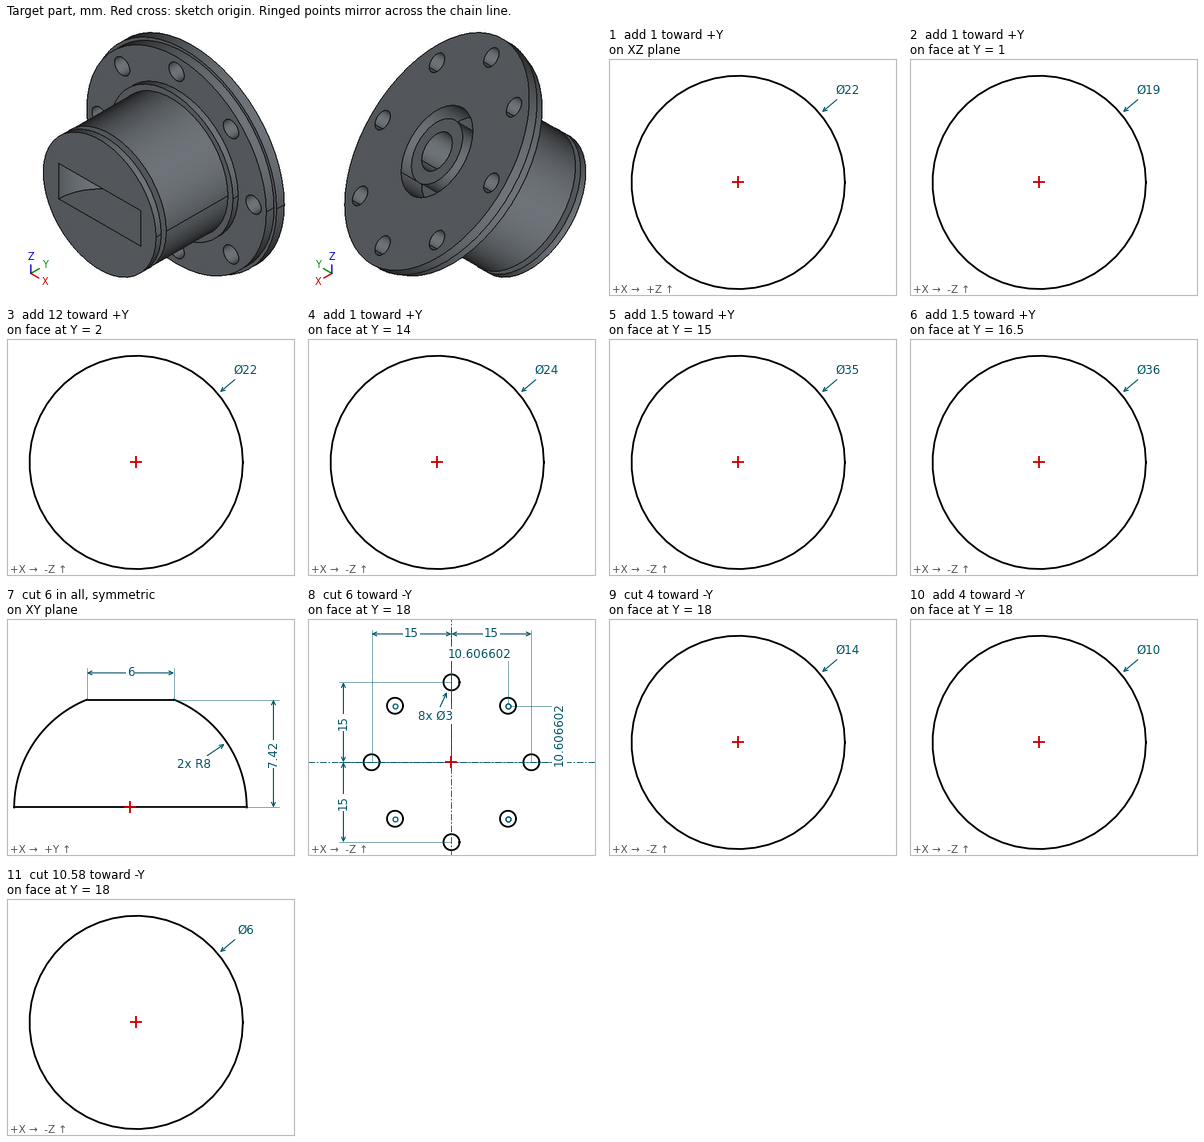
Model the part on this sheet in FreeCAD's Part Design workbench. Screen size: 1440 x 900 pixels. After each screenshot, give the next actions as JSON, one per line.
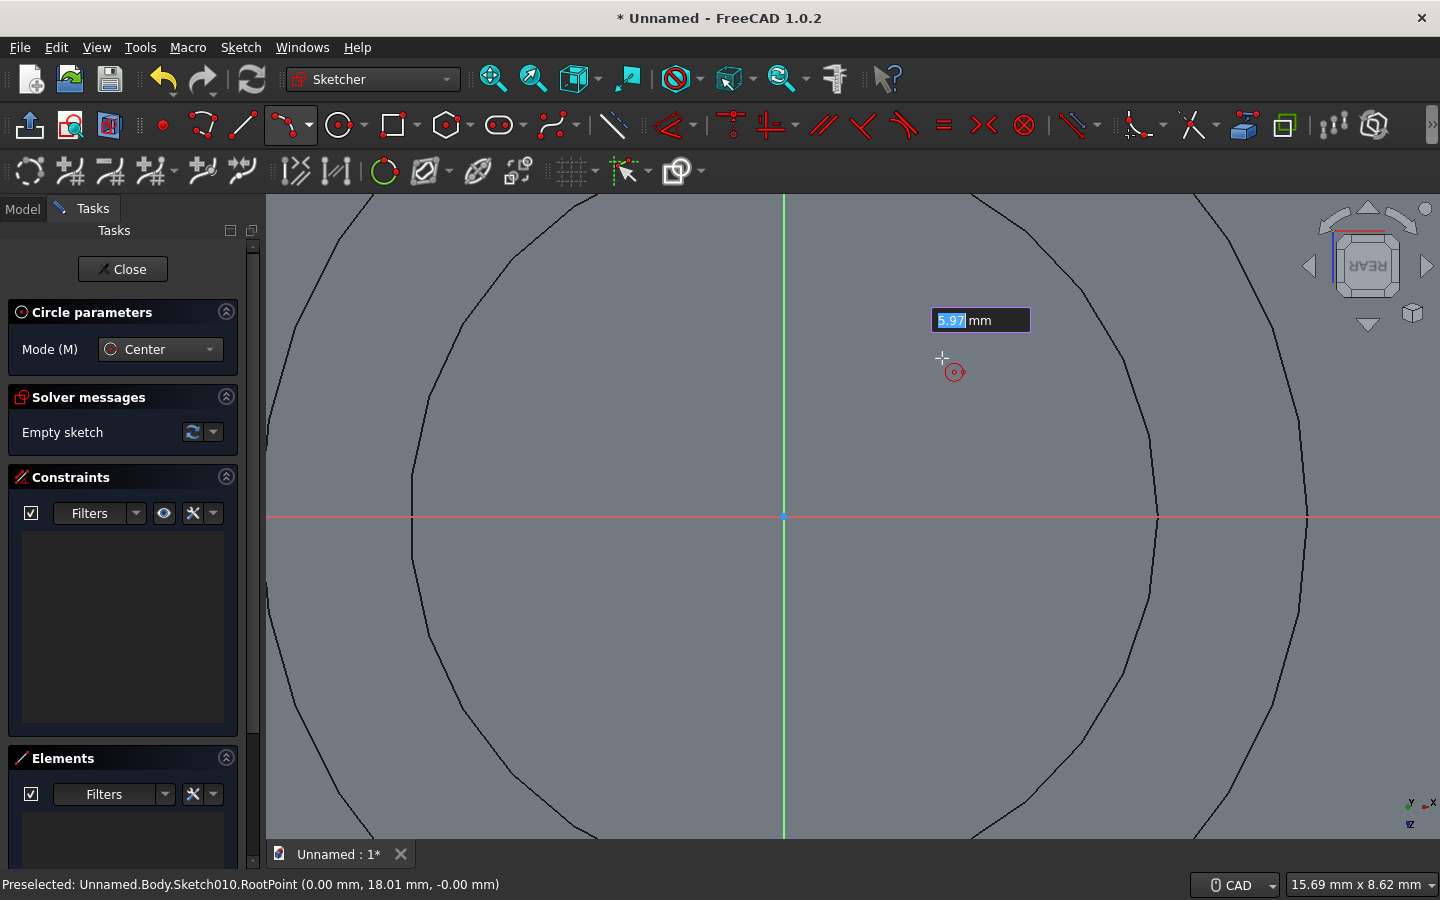
{"action": "type", "text": "6"}
{"action": "key", "text": "Return"}
{"action": "key", "text": "Escape"}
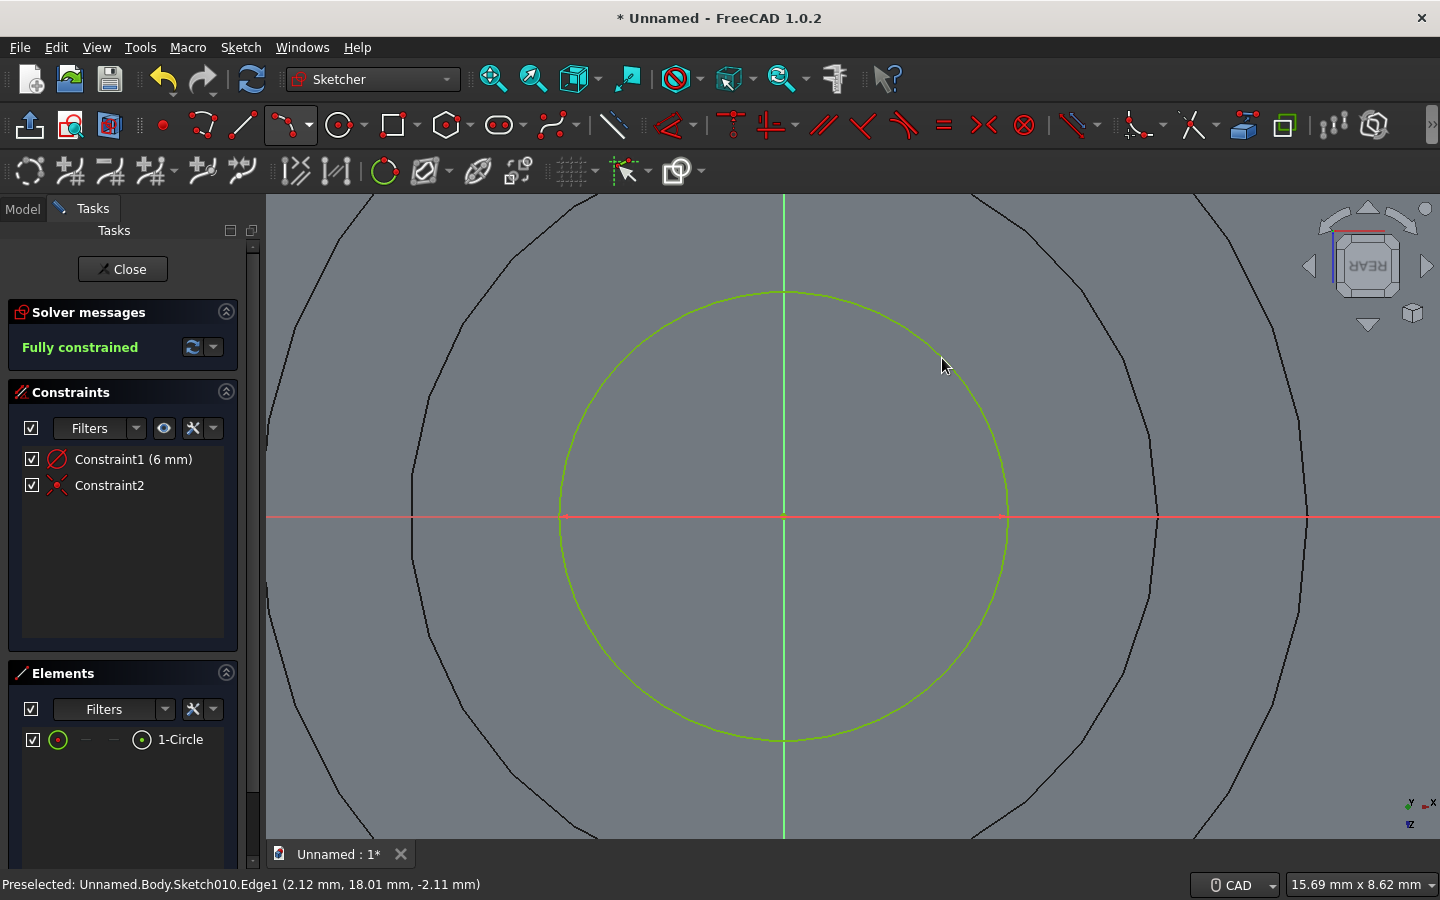
{"action": "left_click", "coordinate": [123, 269]}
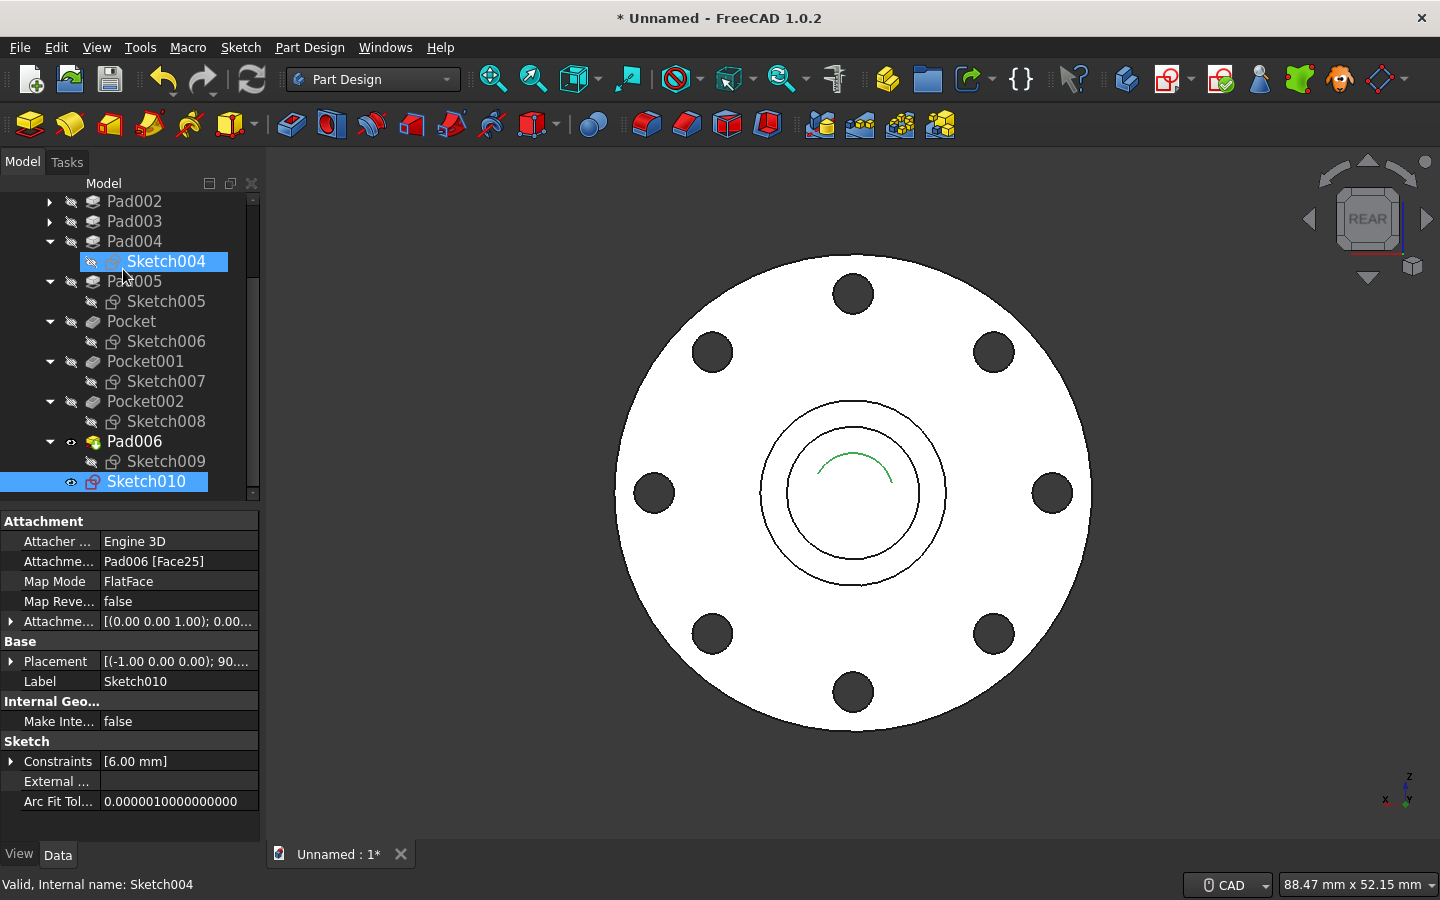
{"action": "left_click", "coordinate": [292, 124]}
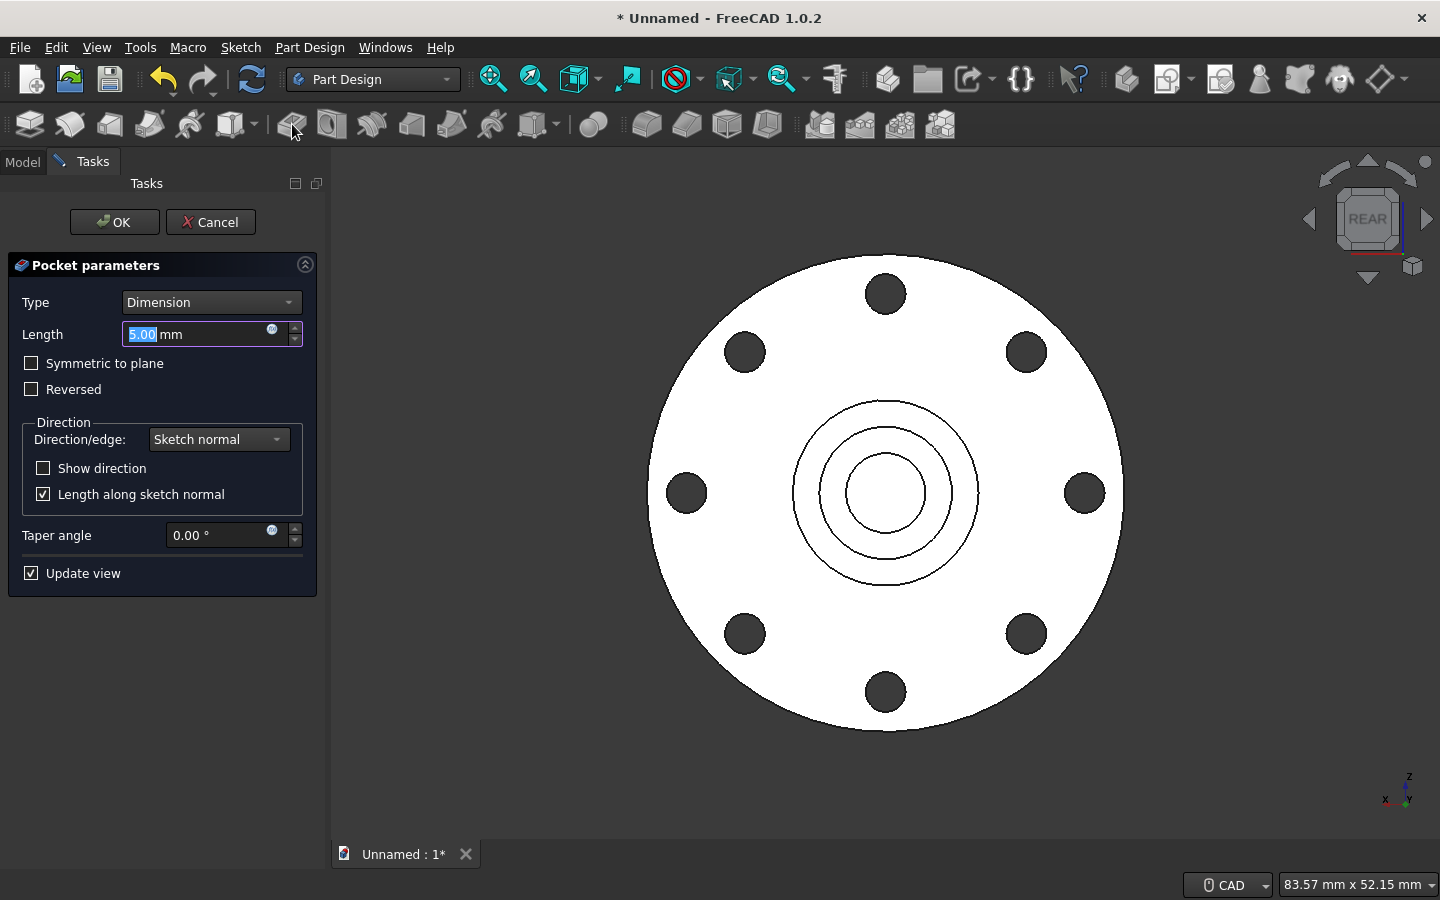
{"action": "type", "text": "10.58"}
{"action": "key", "text": "Tab"}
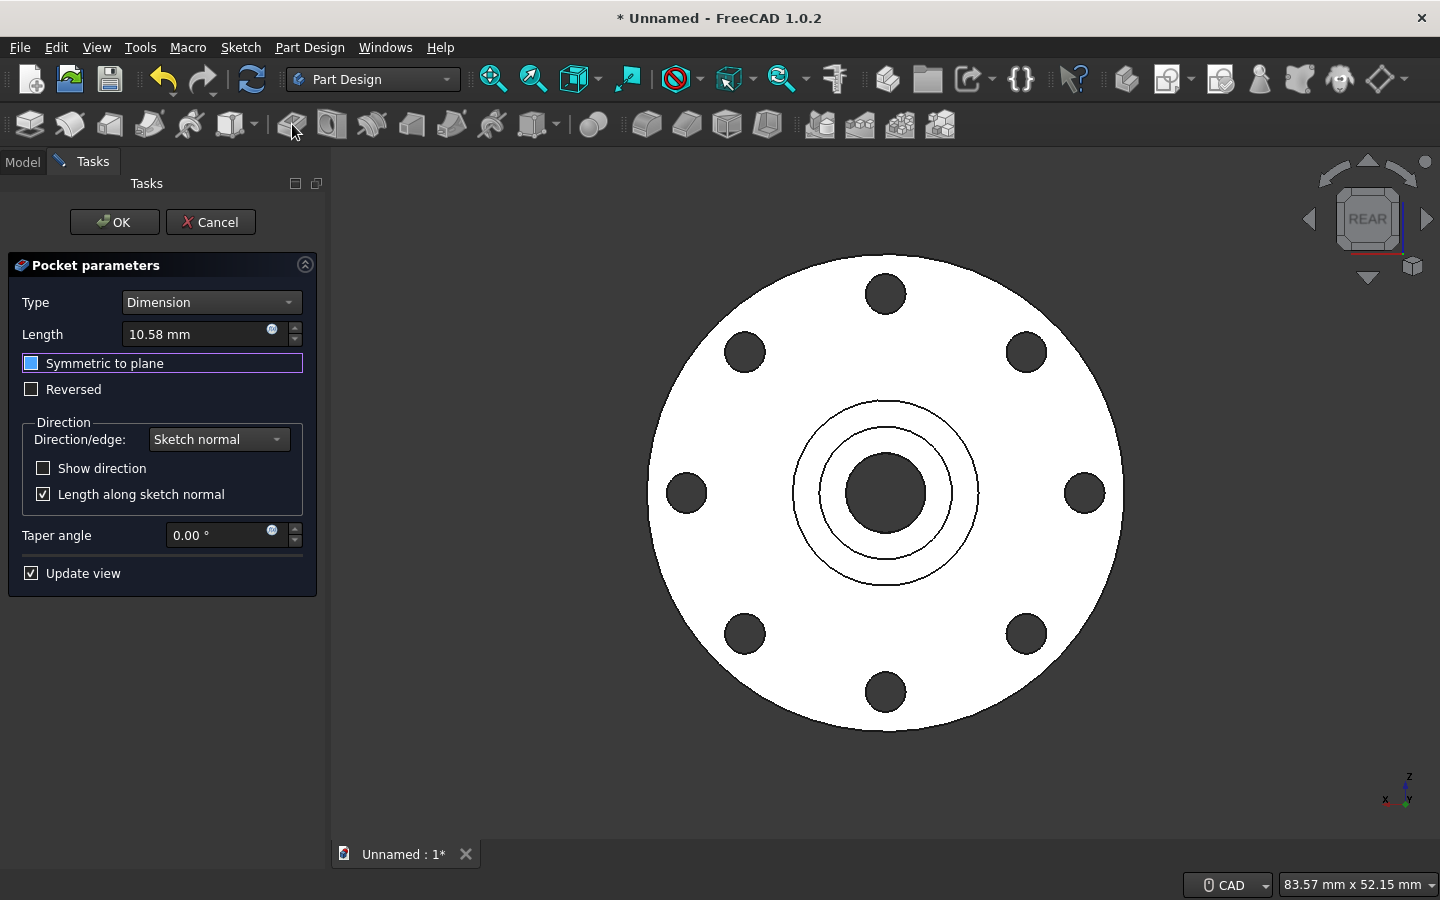
{"action": "left_click", "coordinate": [115, 222]}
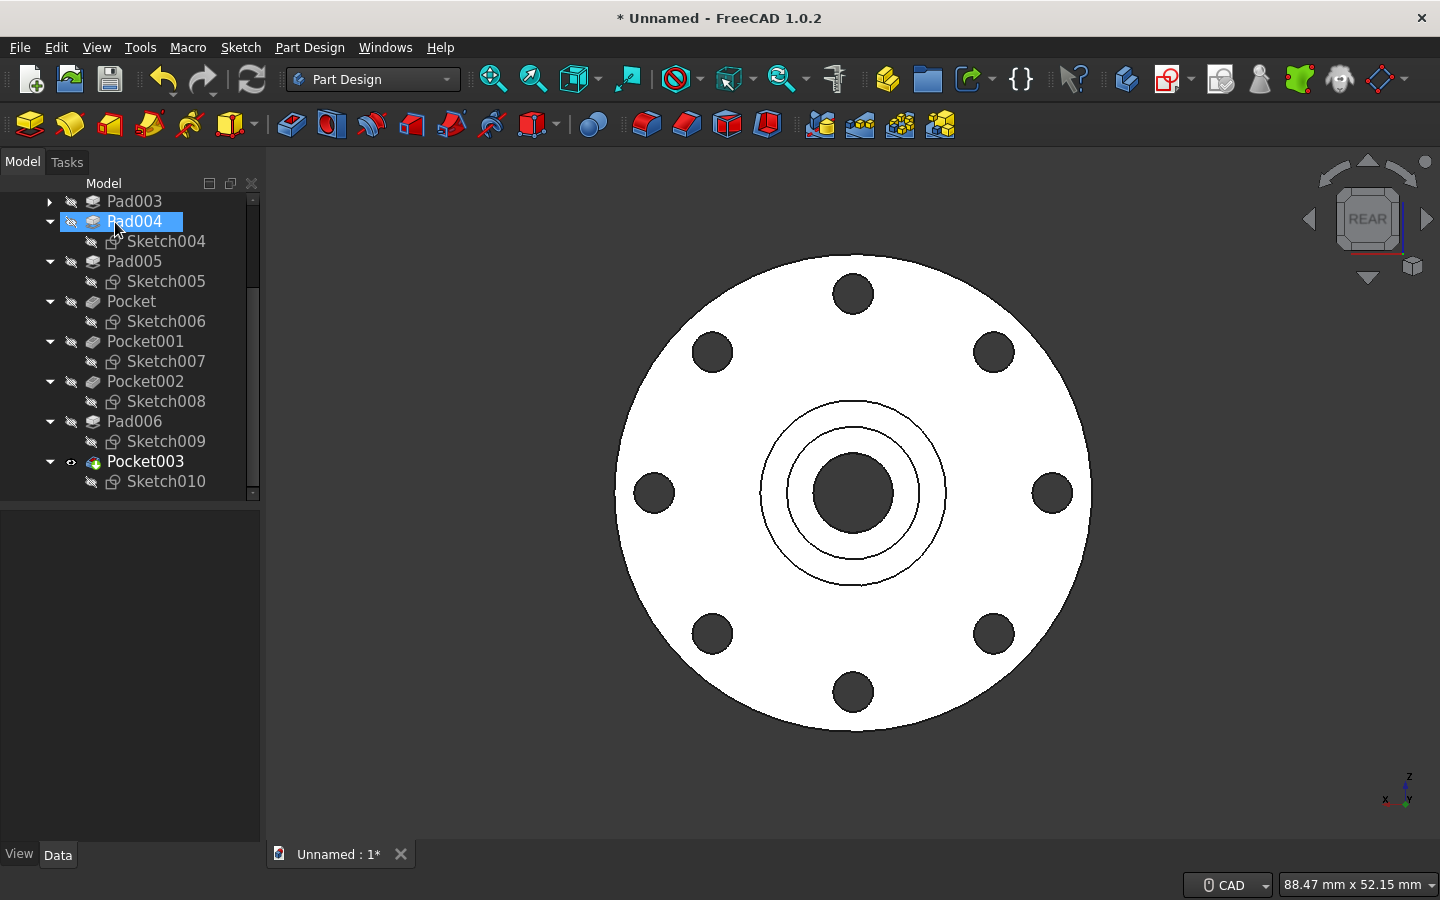
{"action": "key", "text": "0"}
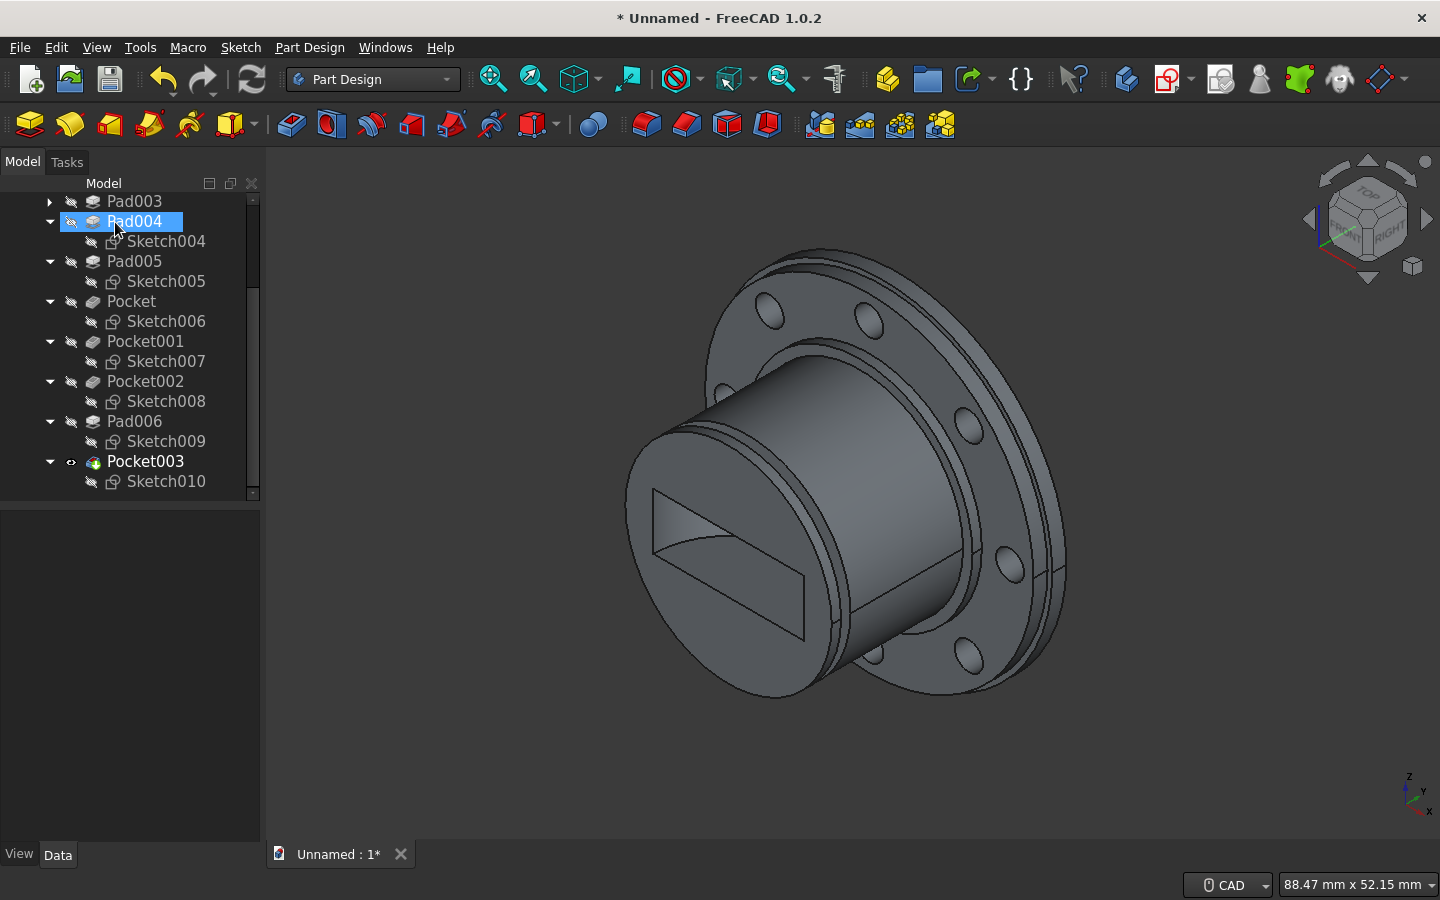
{"action": "left_click", "coordinate": [494, 80]}